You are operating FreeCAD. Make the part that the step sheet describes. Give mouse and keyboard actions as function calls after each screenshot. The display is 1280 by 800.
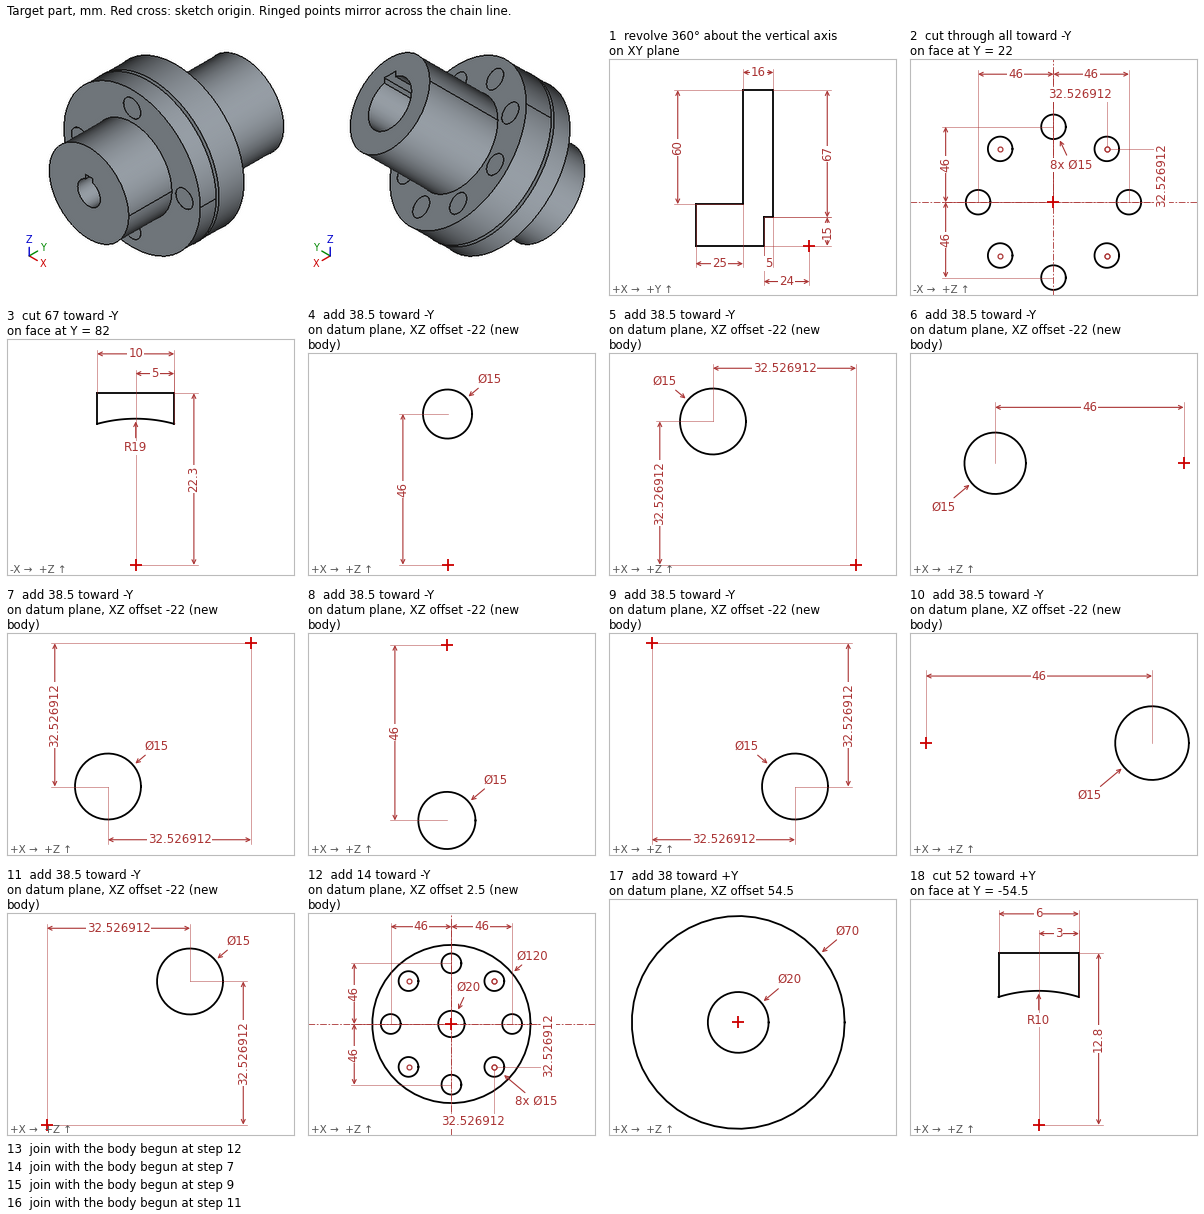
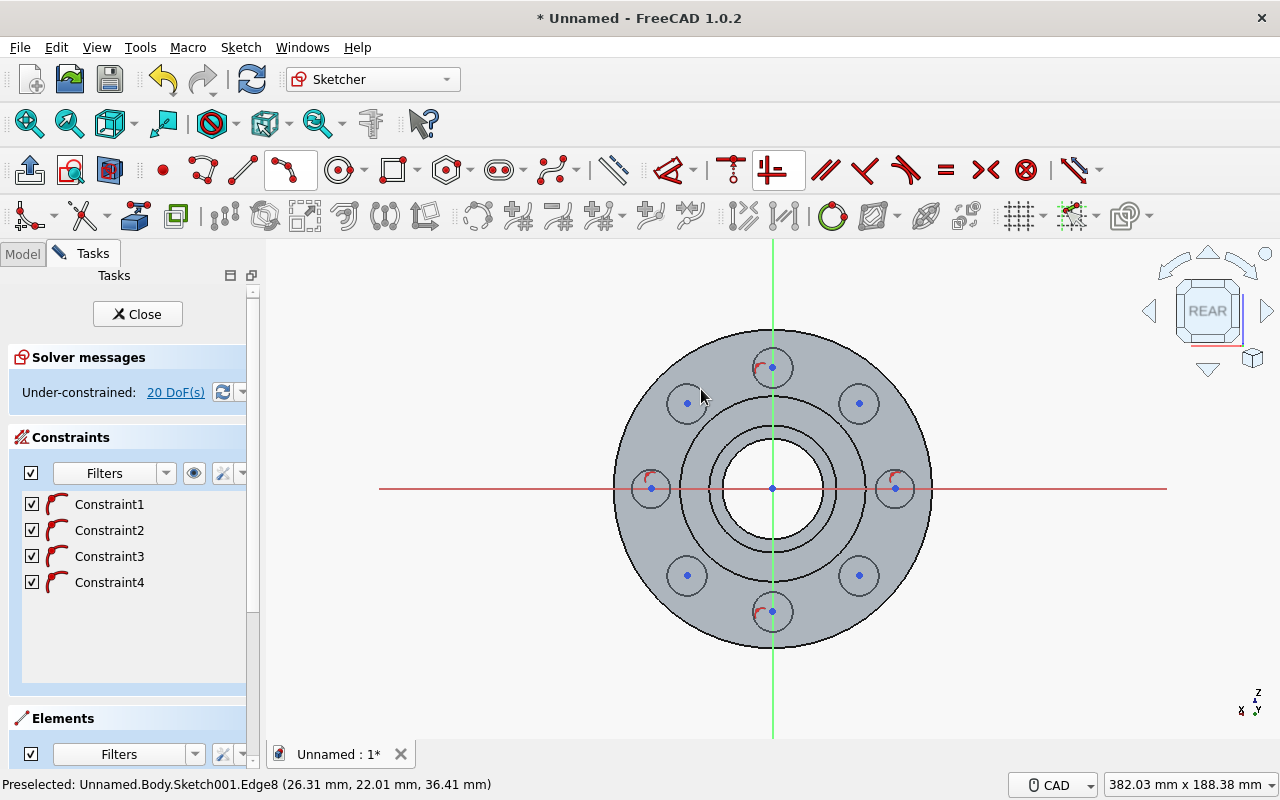
click(787, 354)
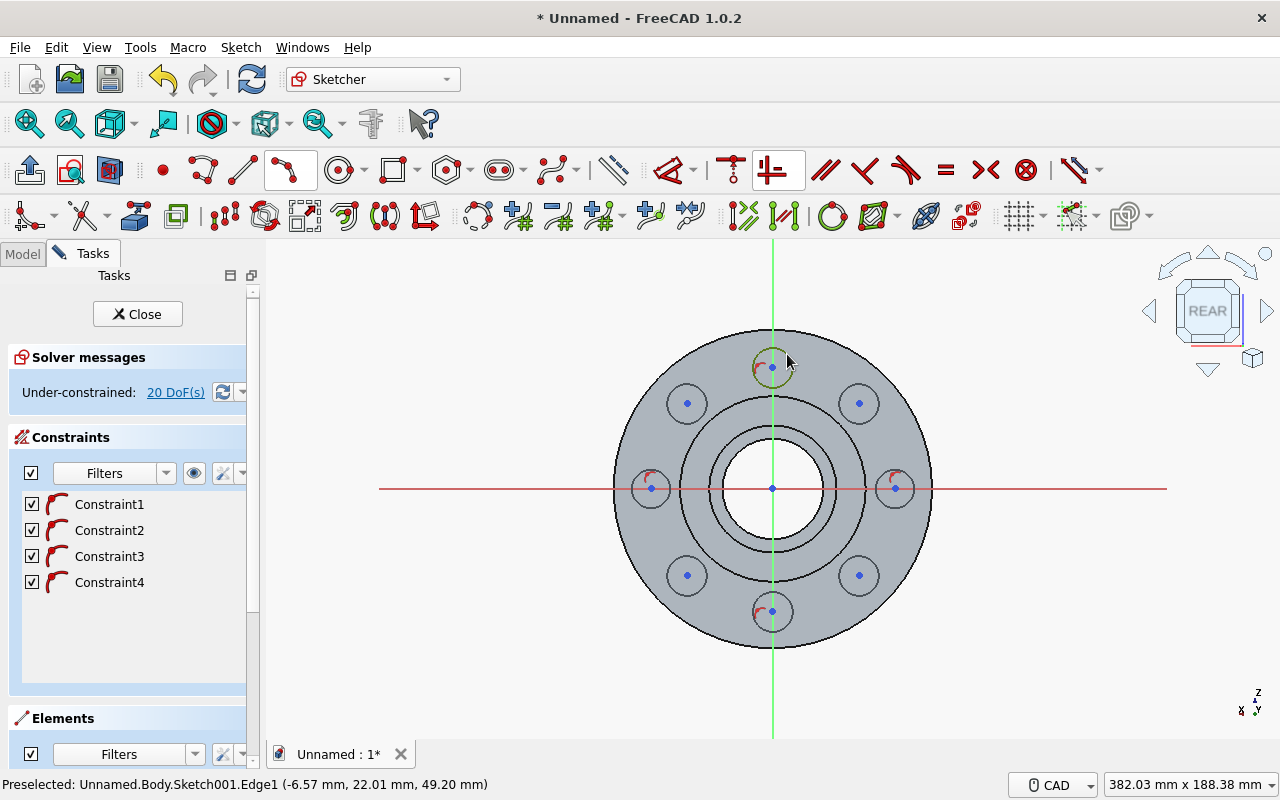
click(873, 390)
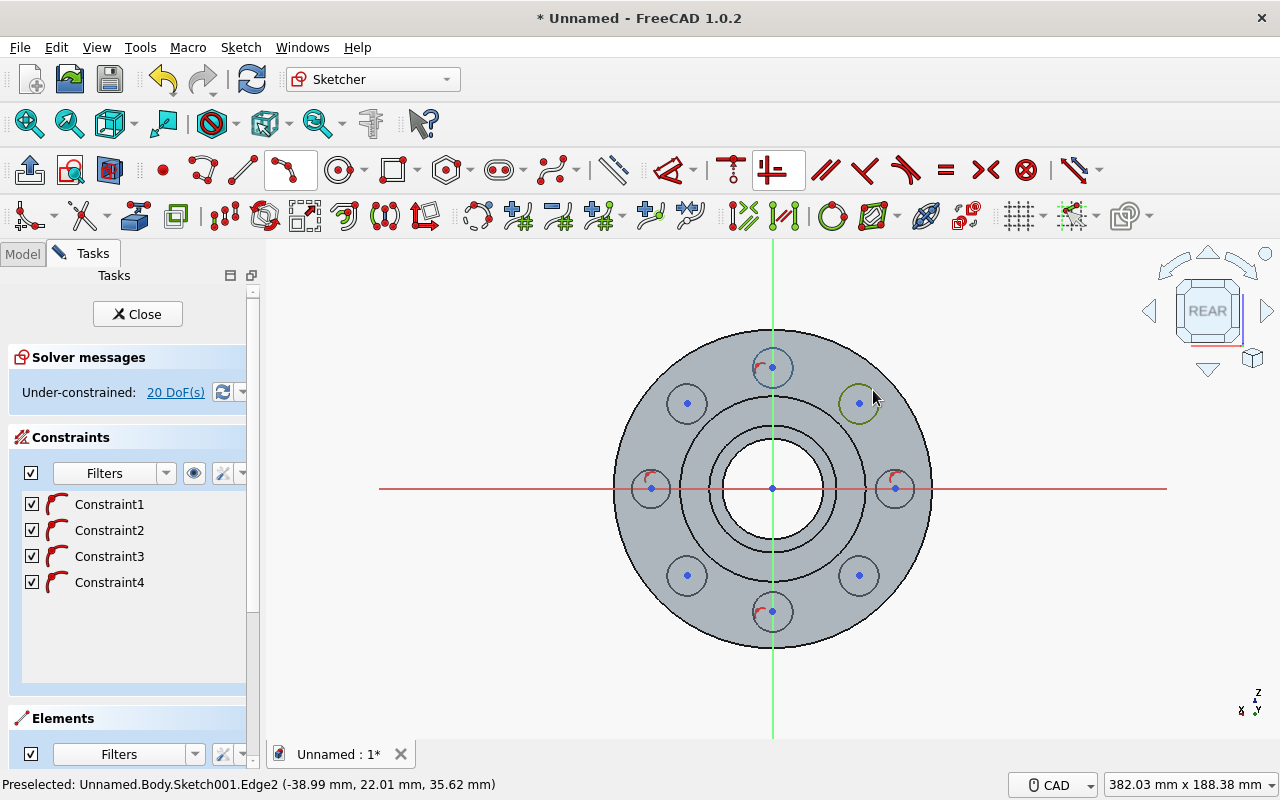
click(908, 475)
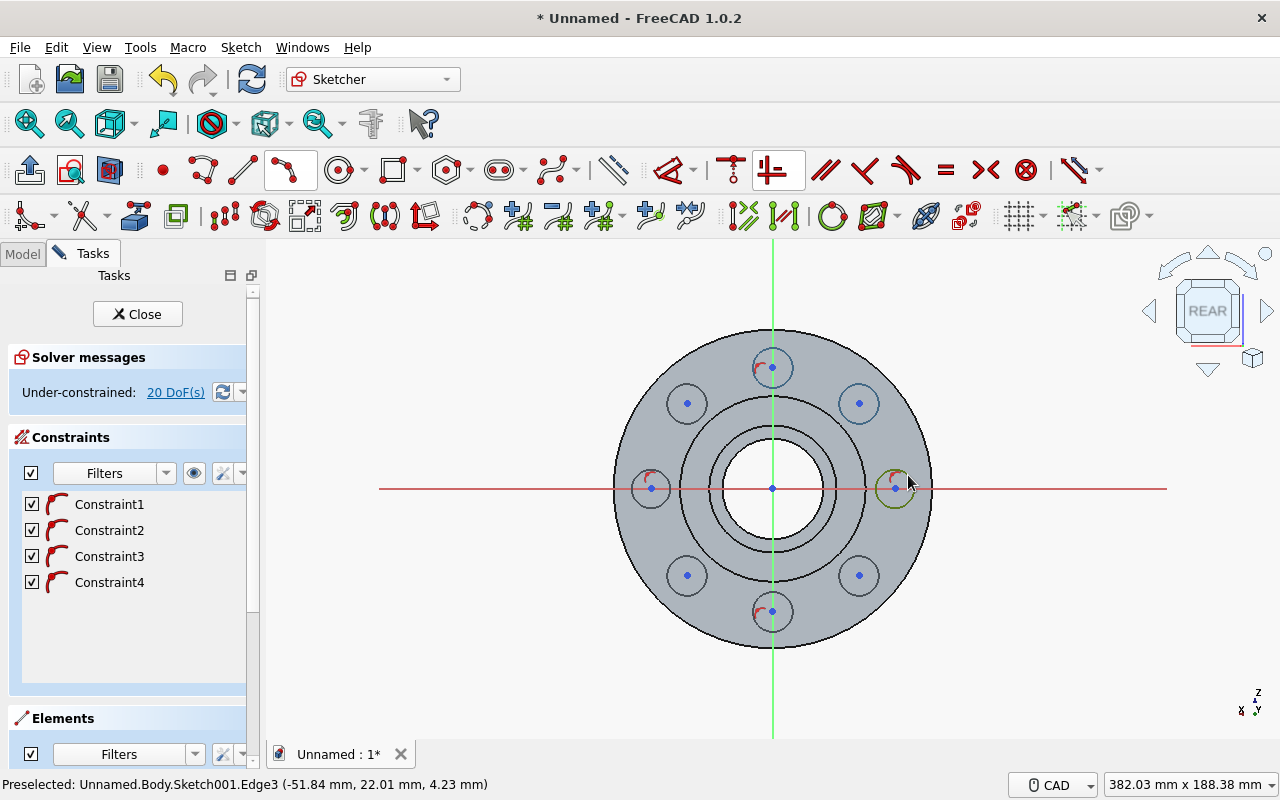
click(873, 562)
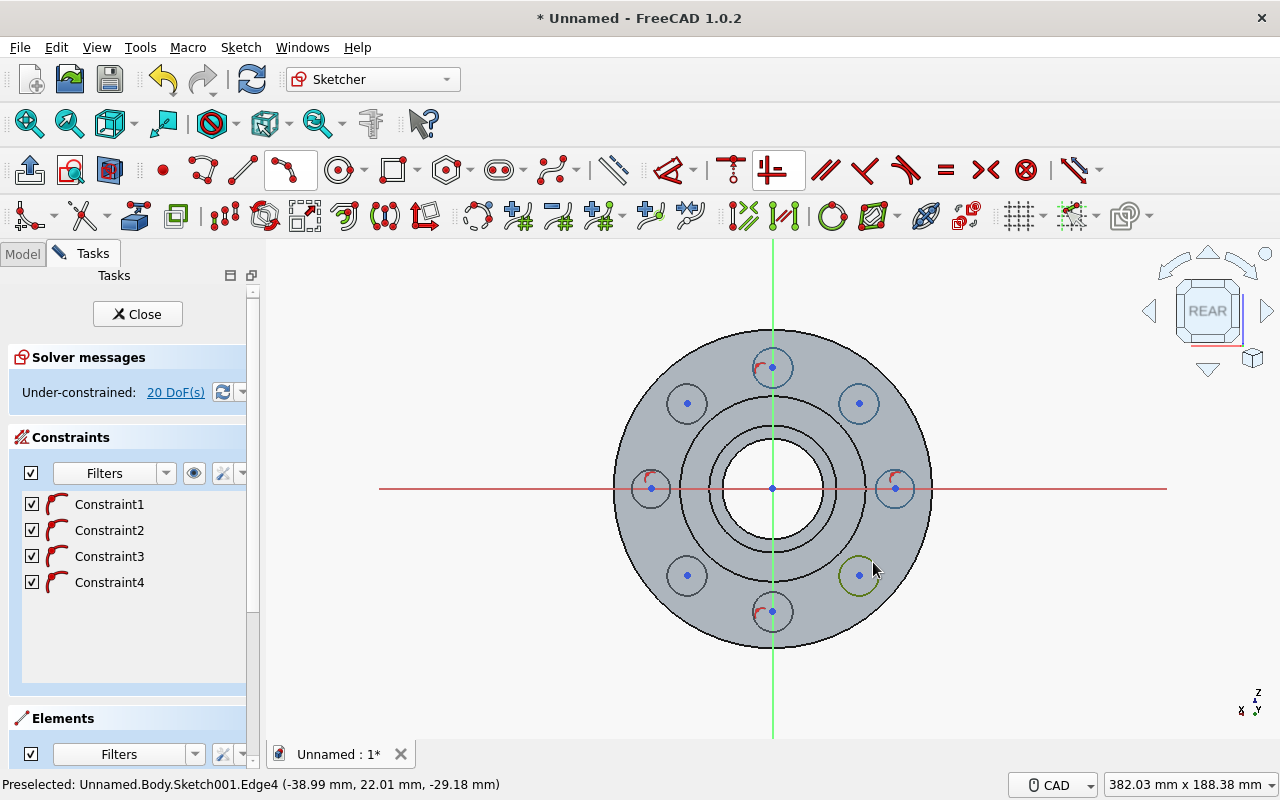
click(787, 598)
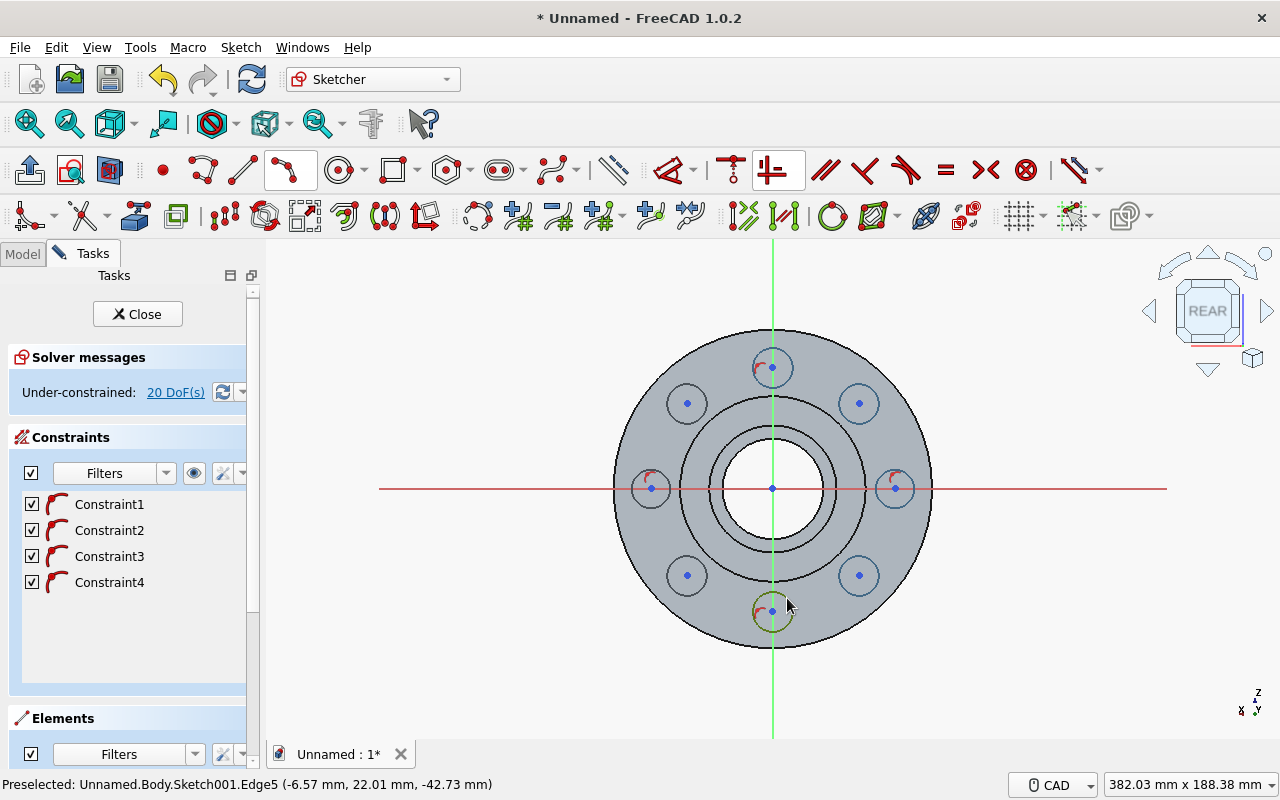
click(701, 562)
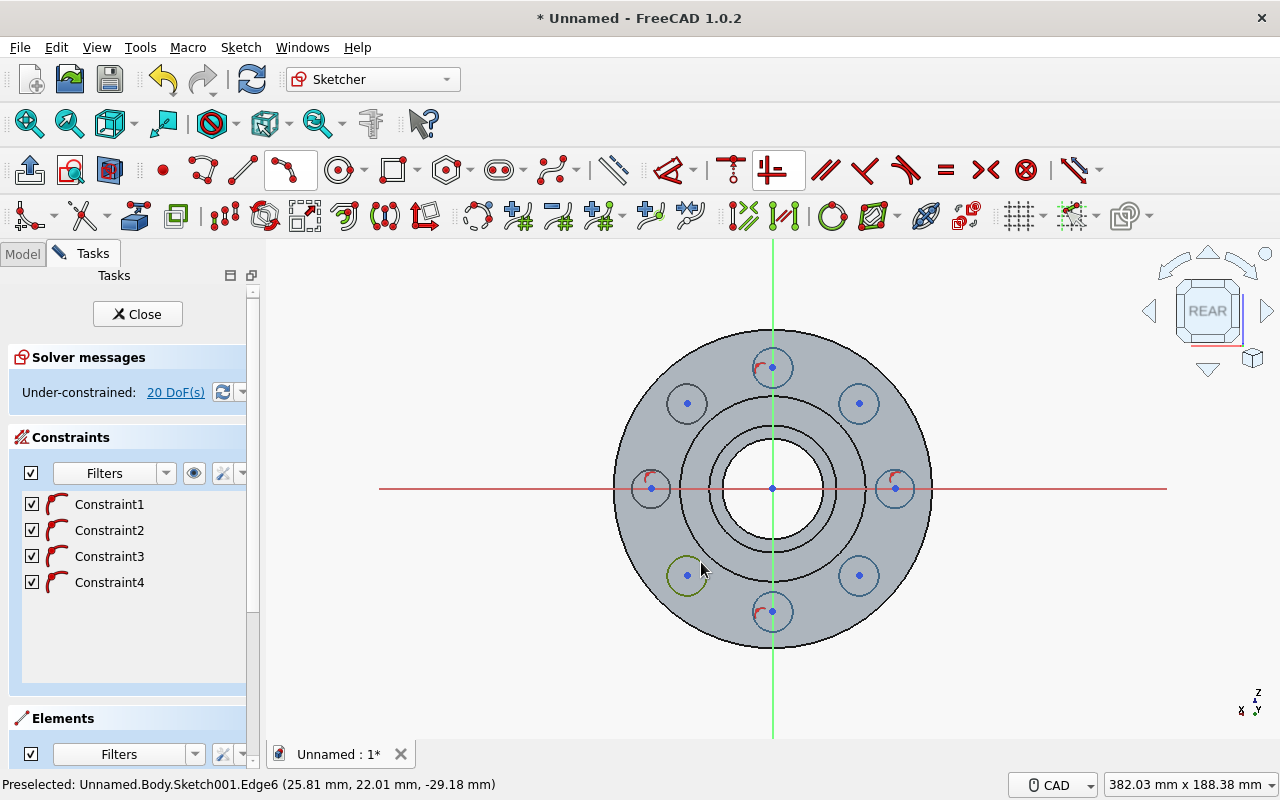
click(664, 475)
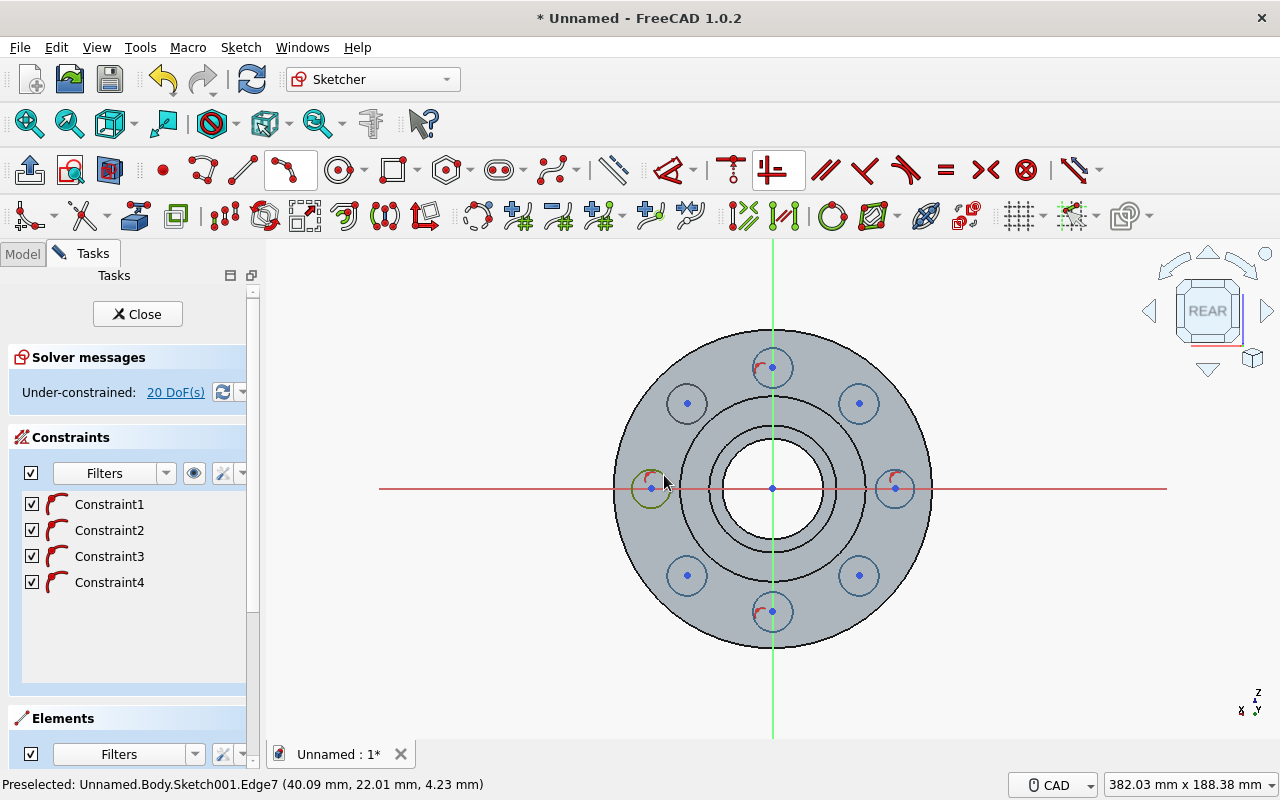
click(701, 390)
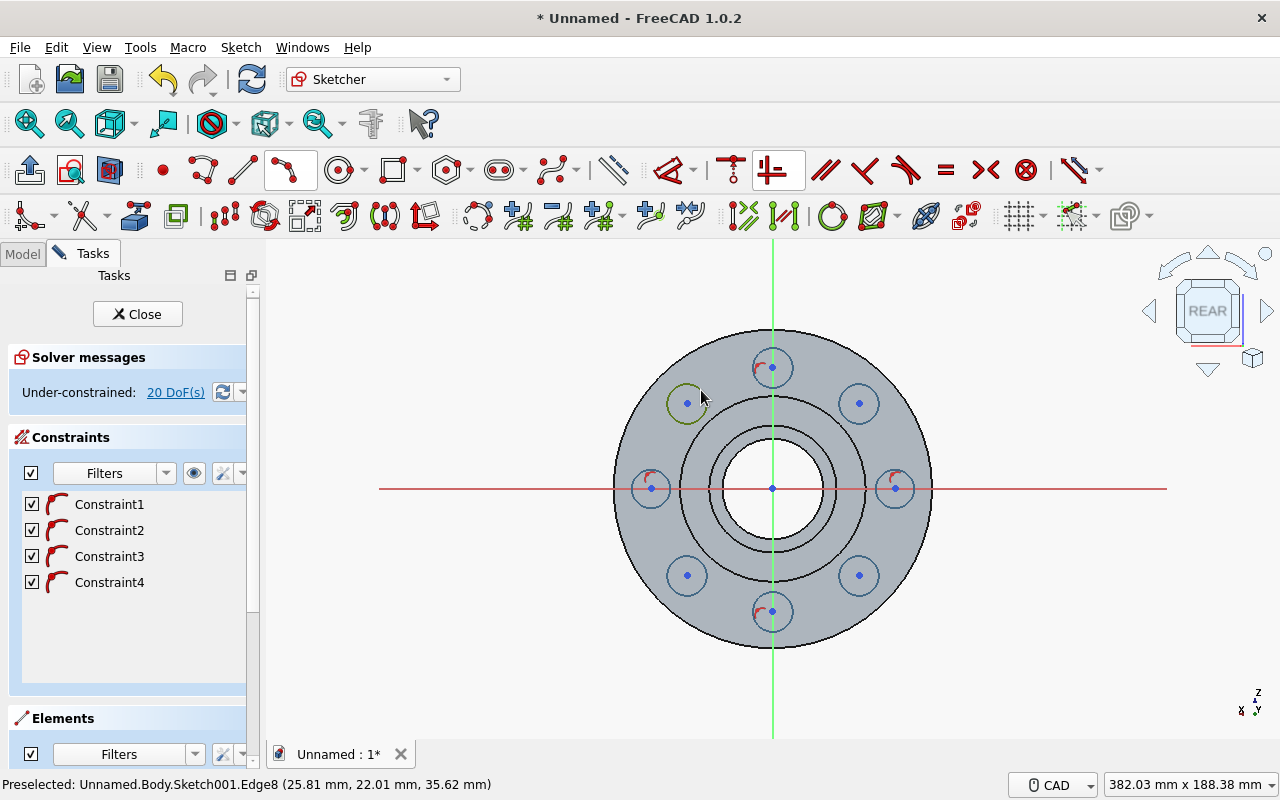
click(946, 170)